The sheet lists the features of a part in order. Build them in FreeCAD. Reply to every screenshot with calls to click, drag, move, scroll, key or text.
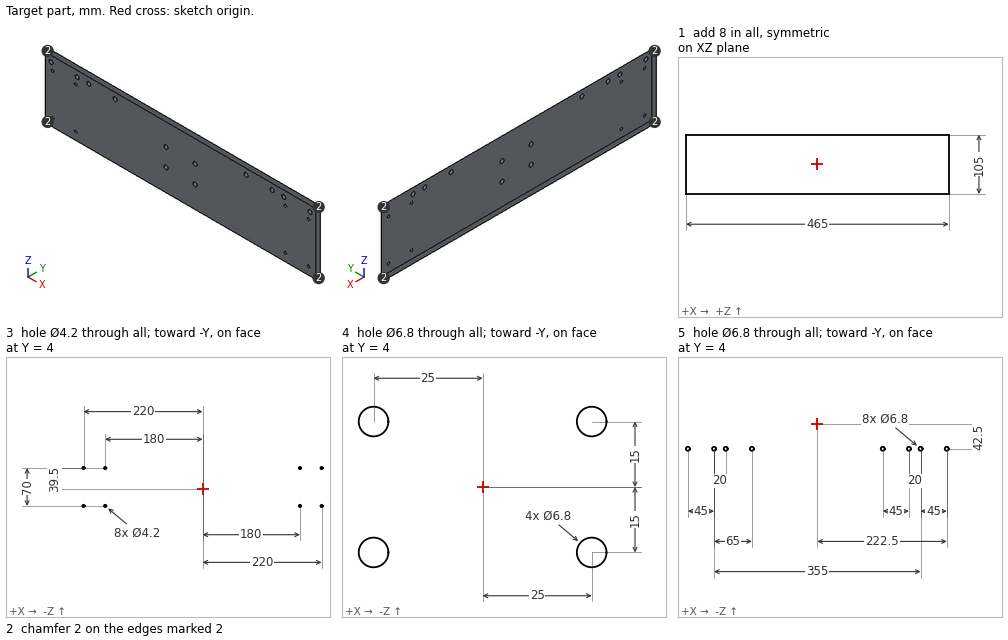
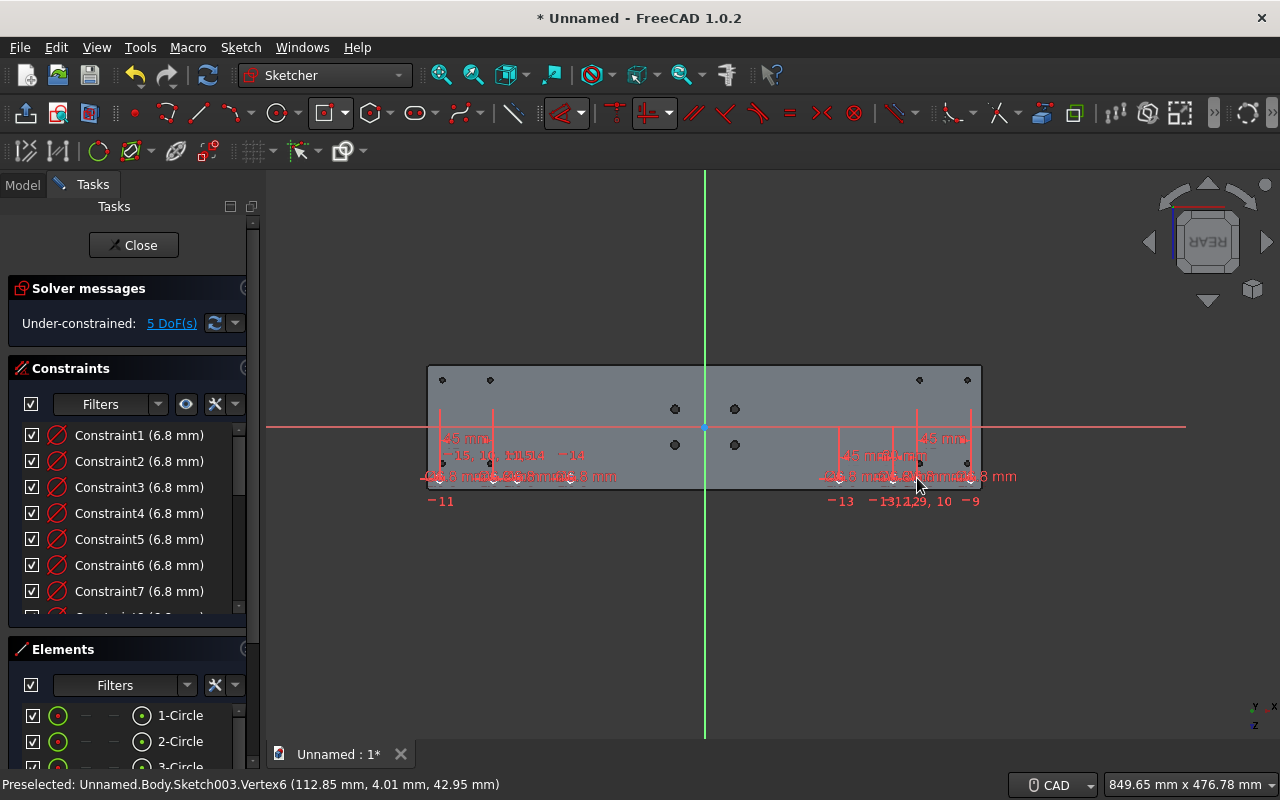
click(493, 479)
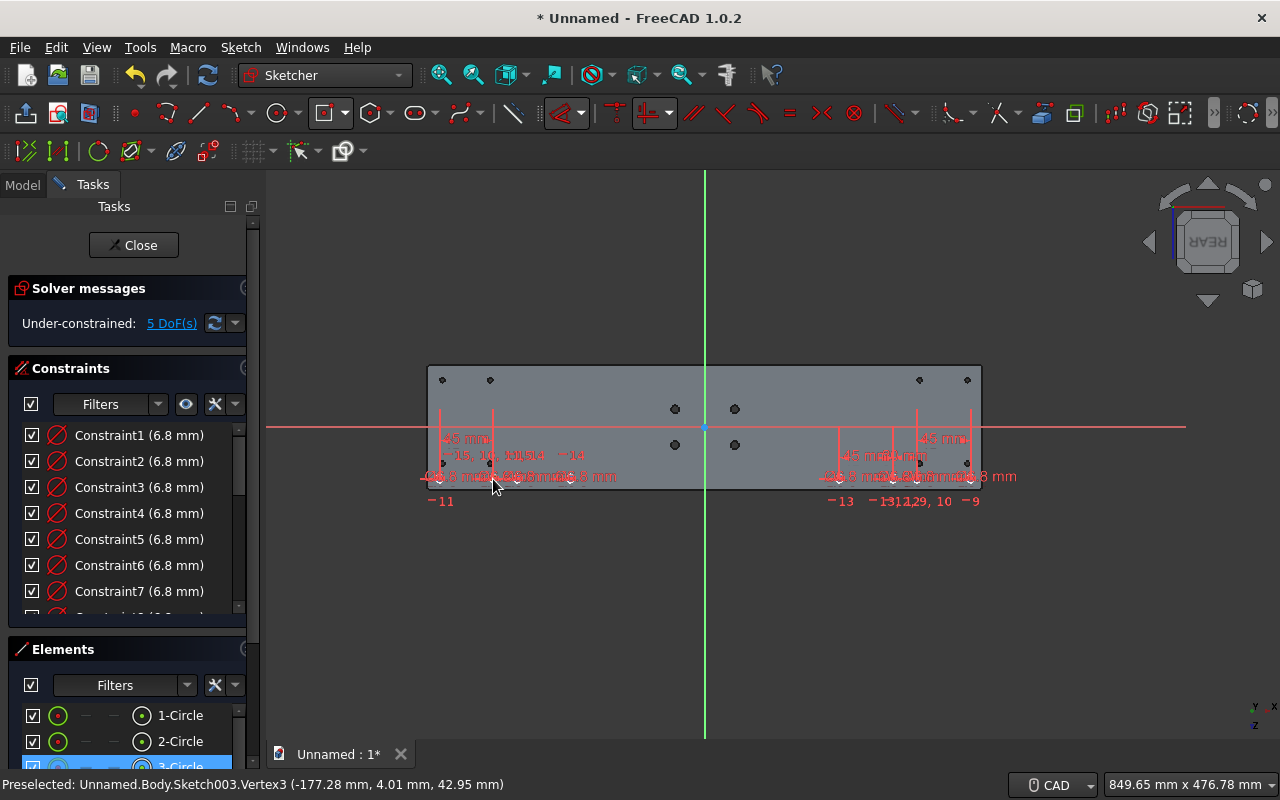
click(570, 479)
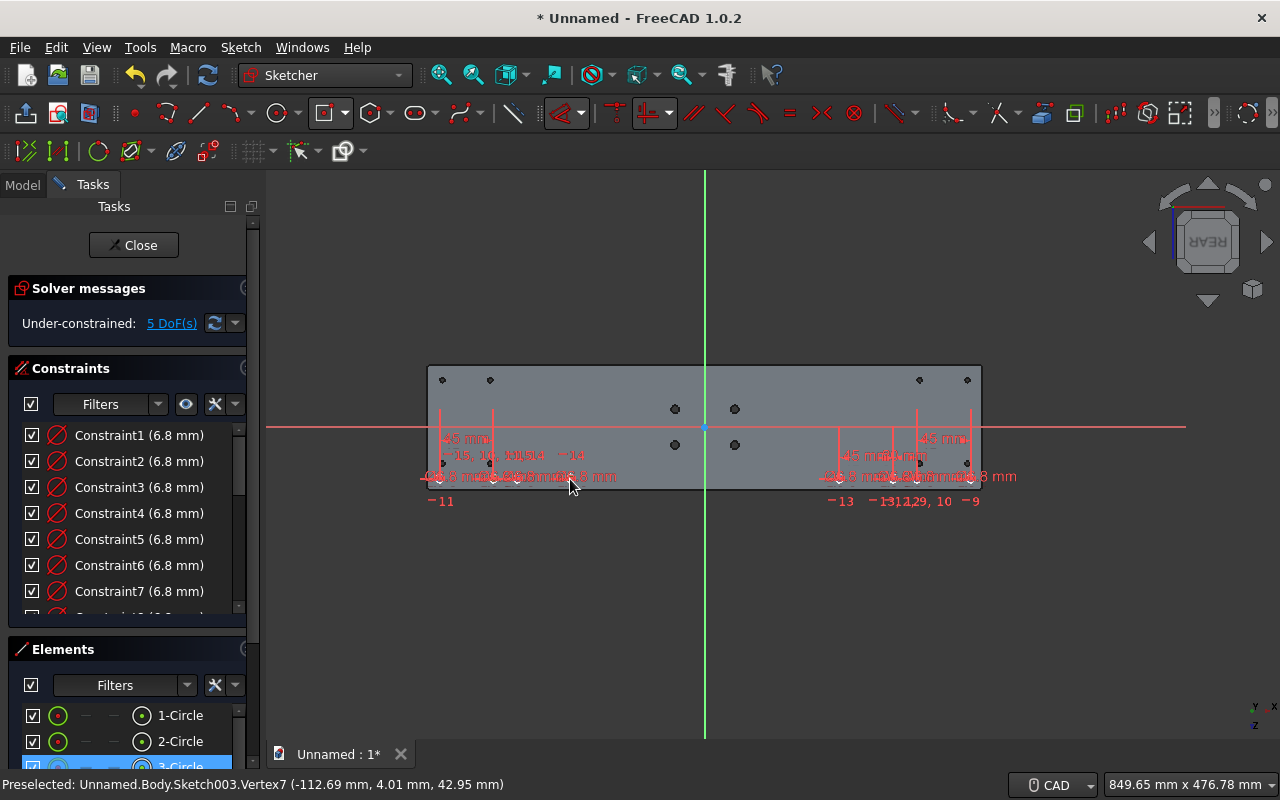
click(584, 114)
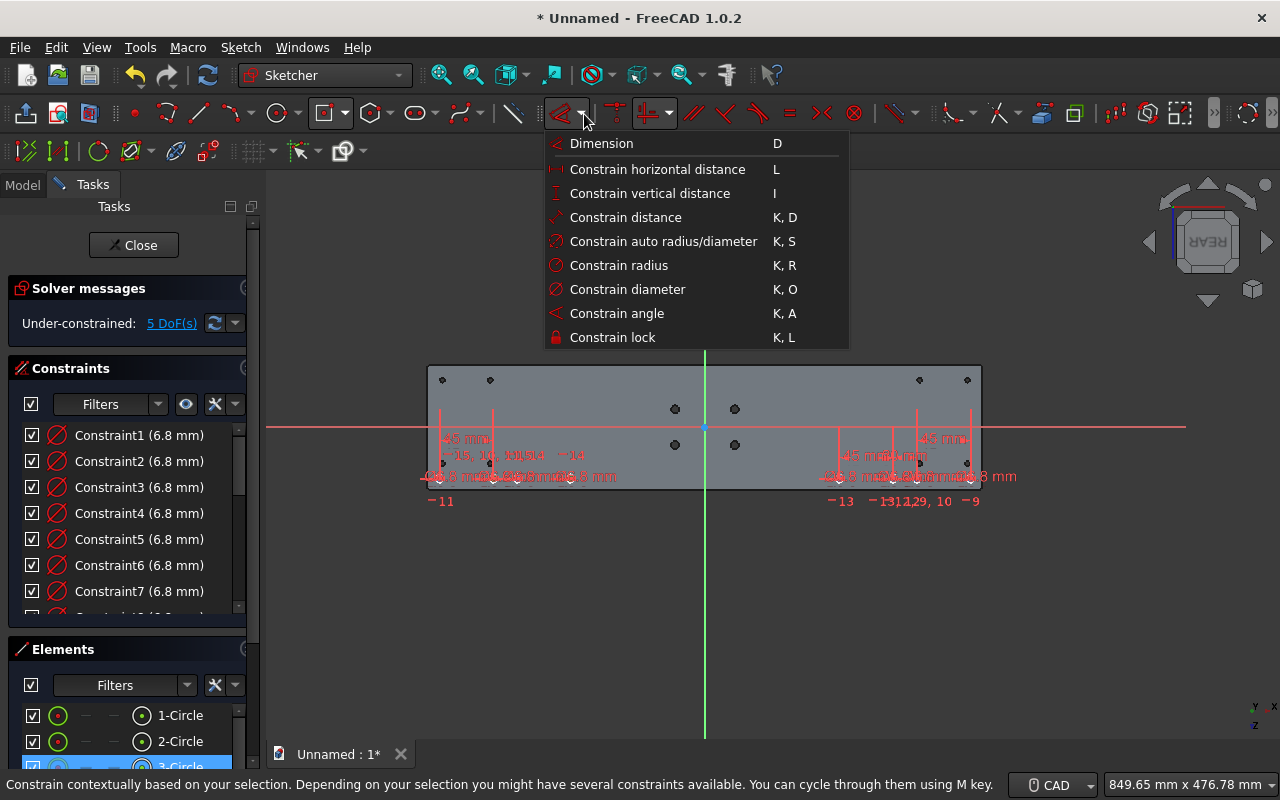
click(697, 169)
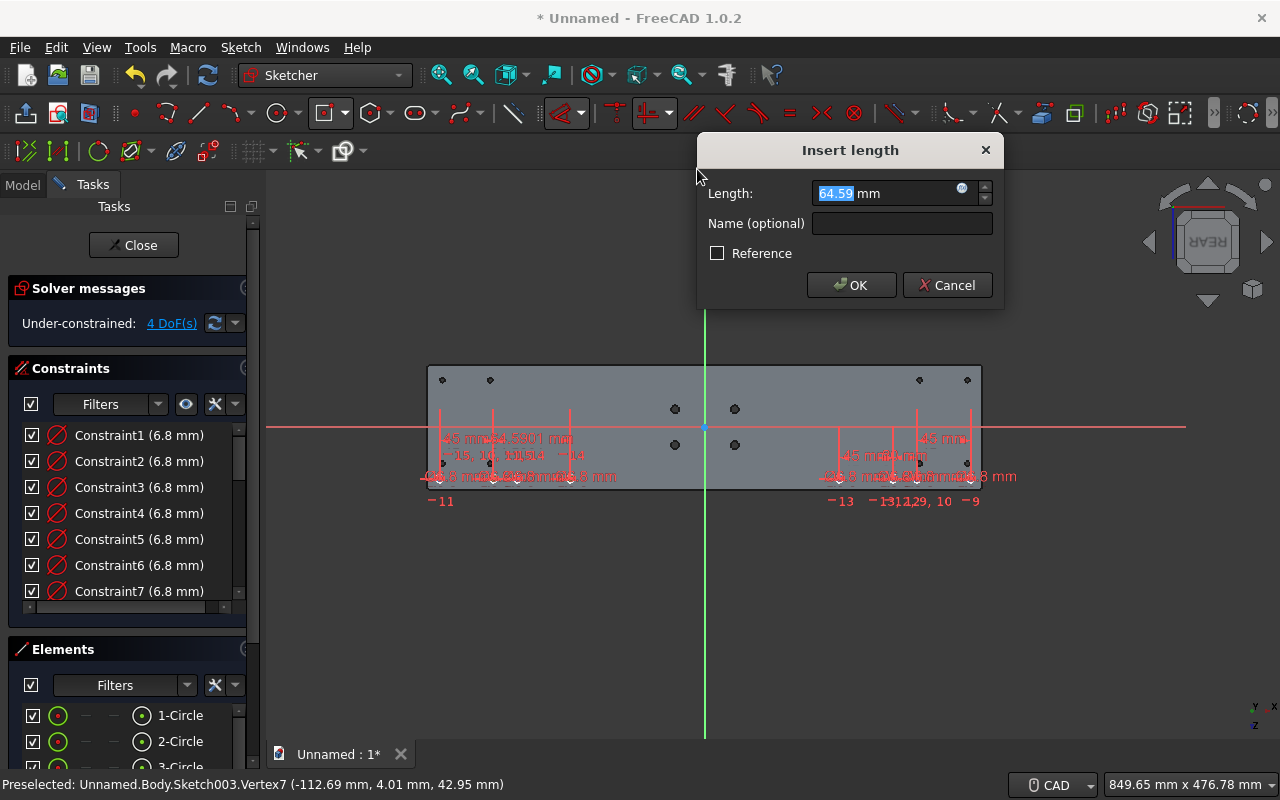
text(65)
key(Return)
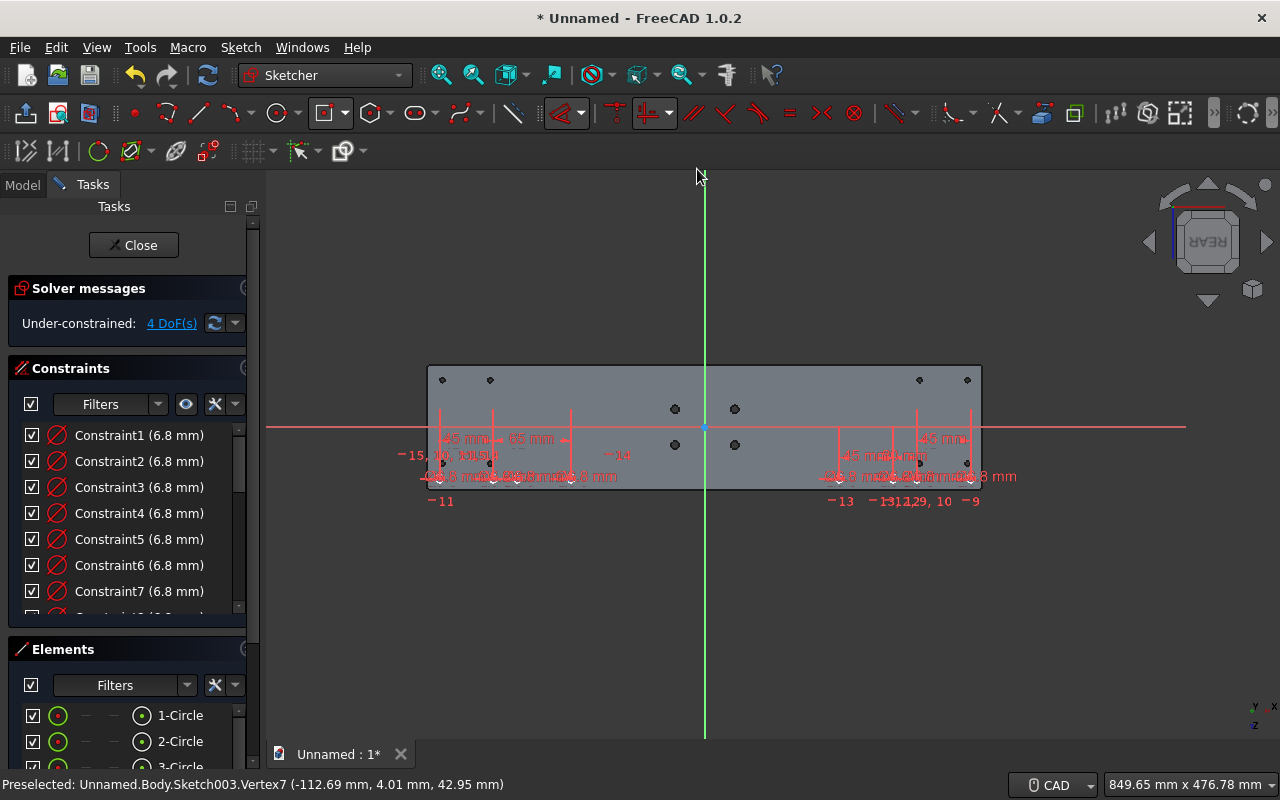
scroll(493, 479, up, 3)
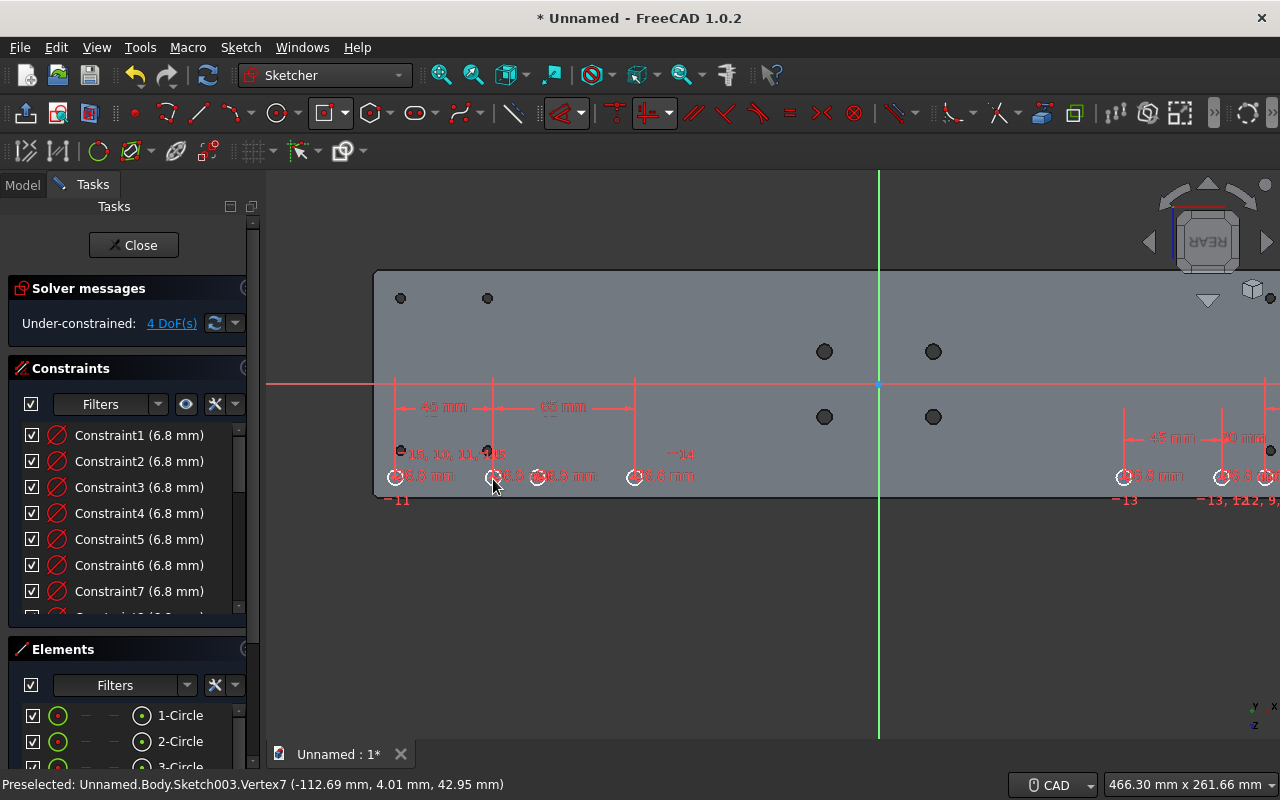
click(493, 478)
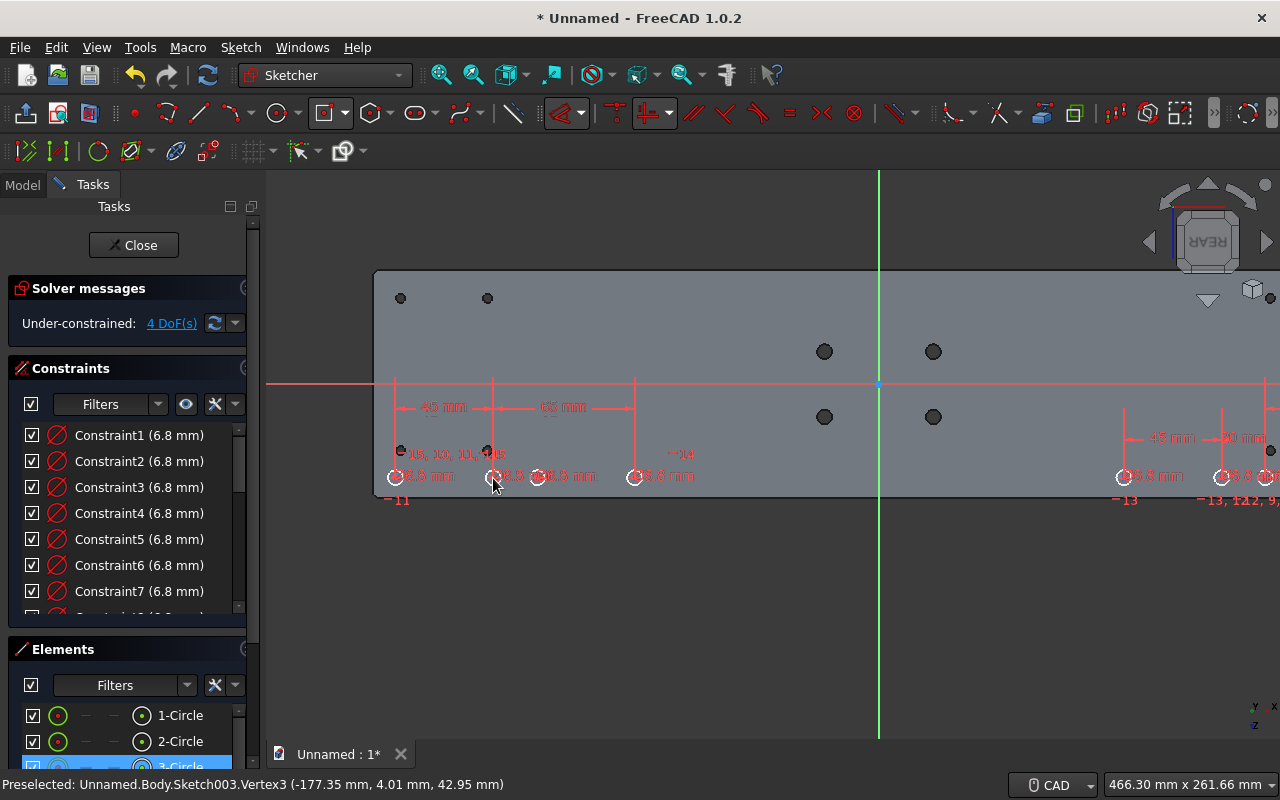
click(537, 478)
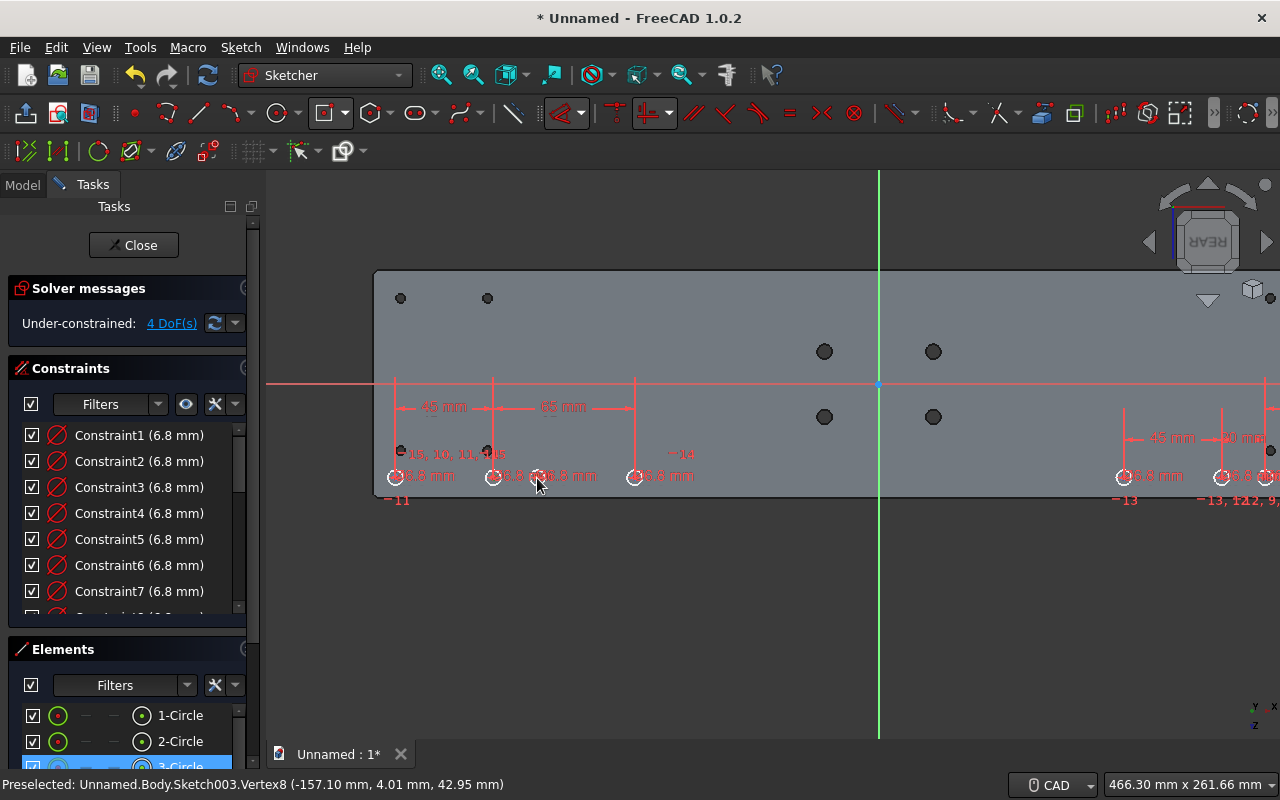
click(584, 114)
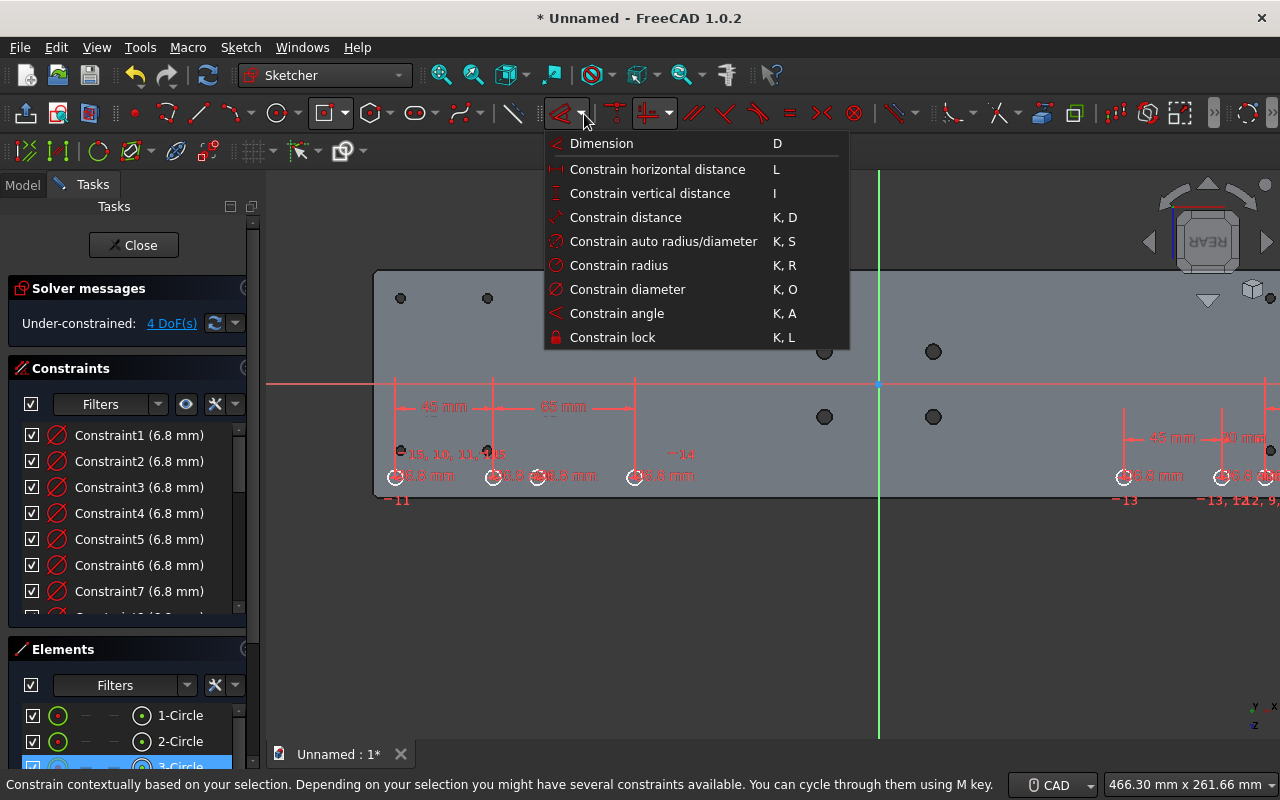
click(697, 169)